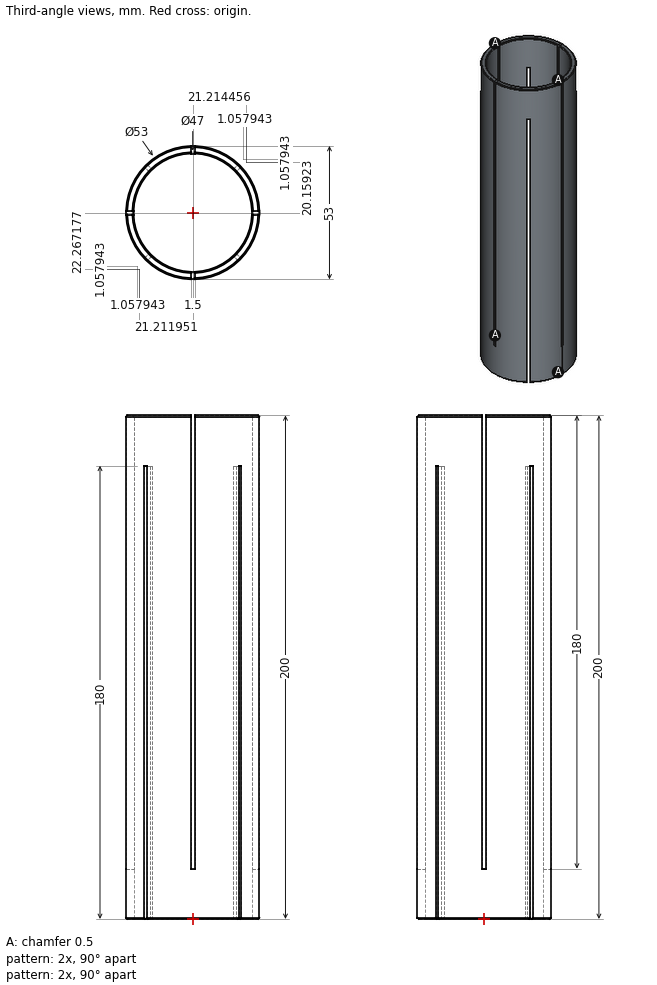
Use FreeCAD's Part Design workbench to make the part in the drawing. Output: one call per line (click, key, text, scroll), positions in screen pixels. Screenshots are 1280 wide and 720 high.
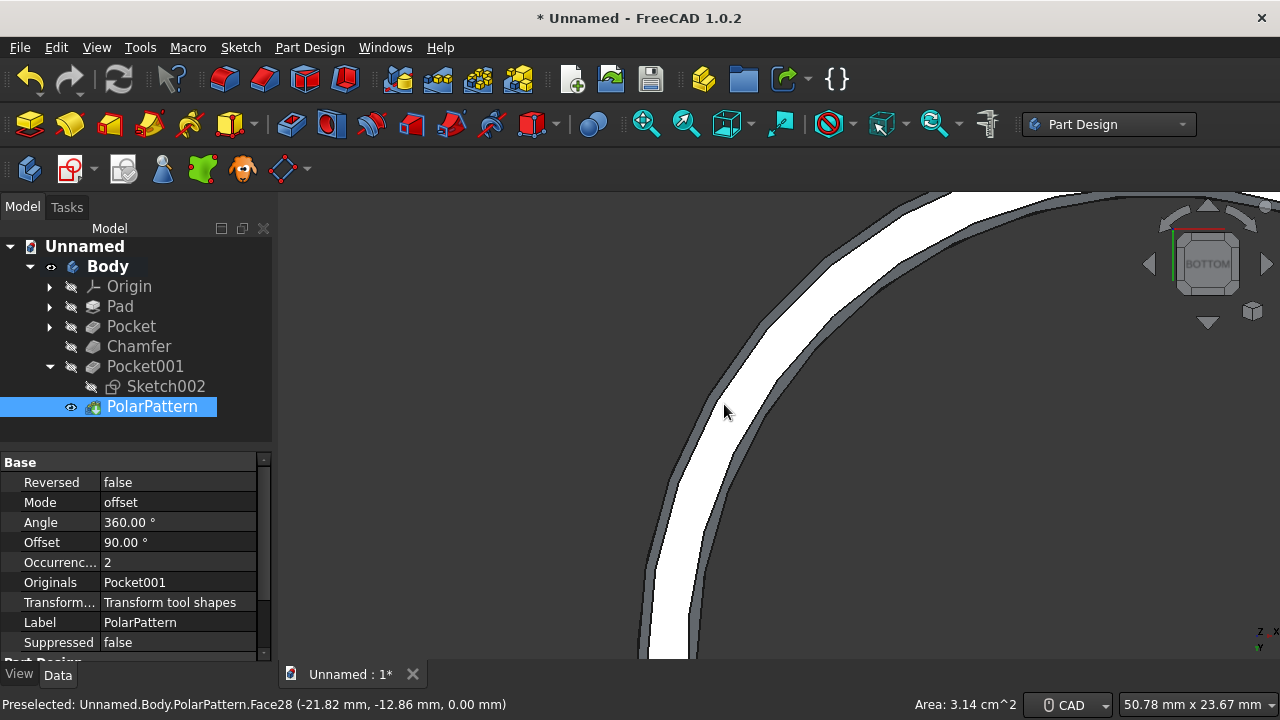
click(70, 170)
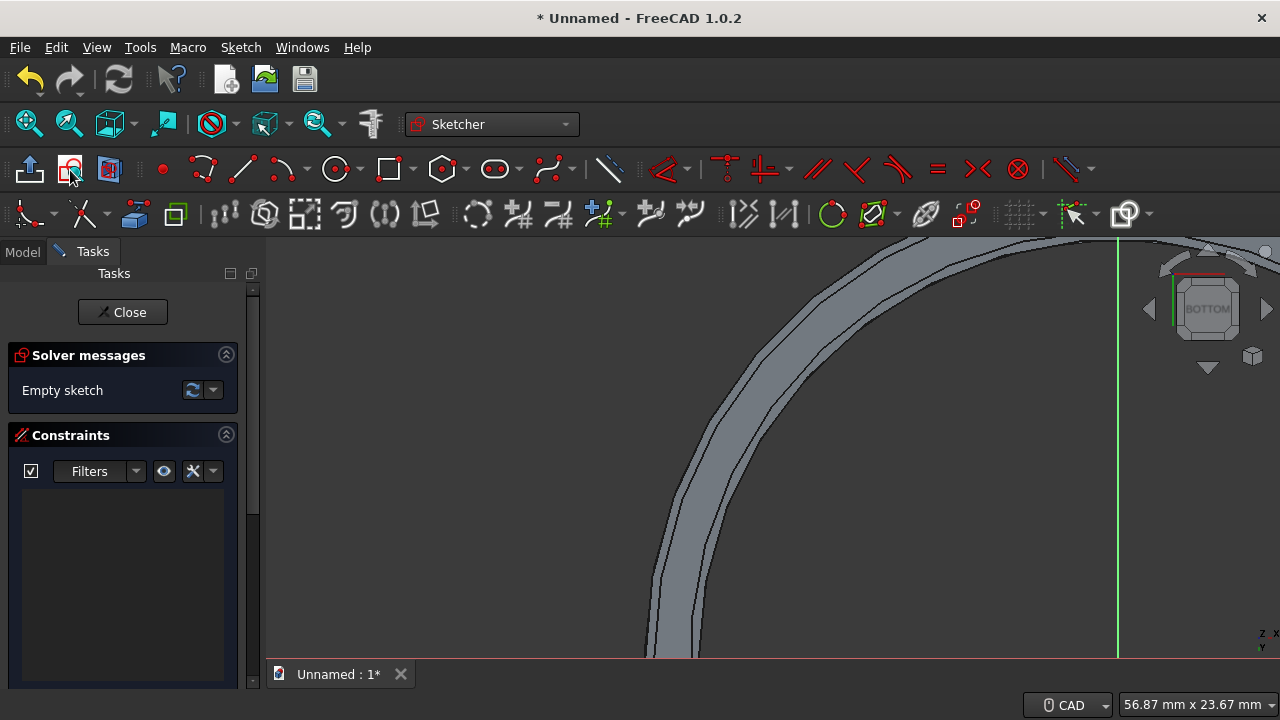
scroll(469, 331, down, 5)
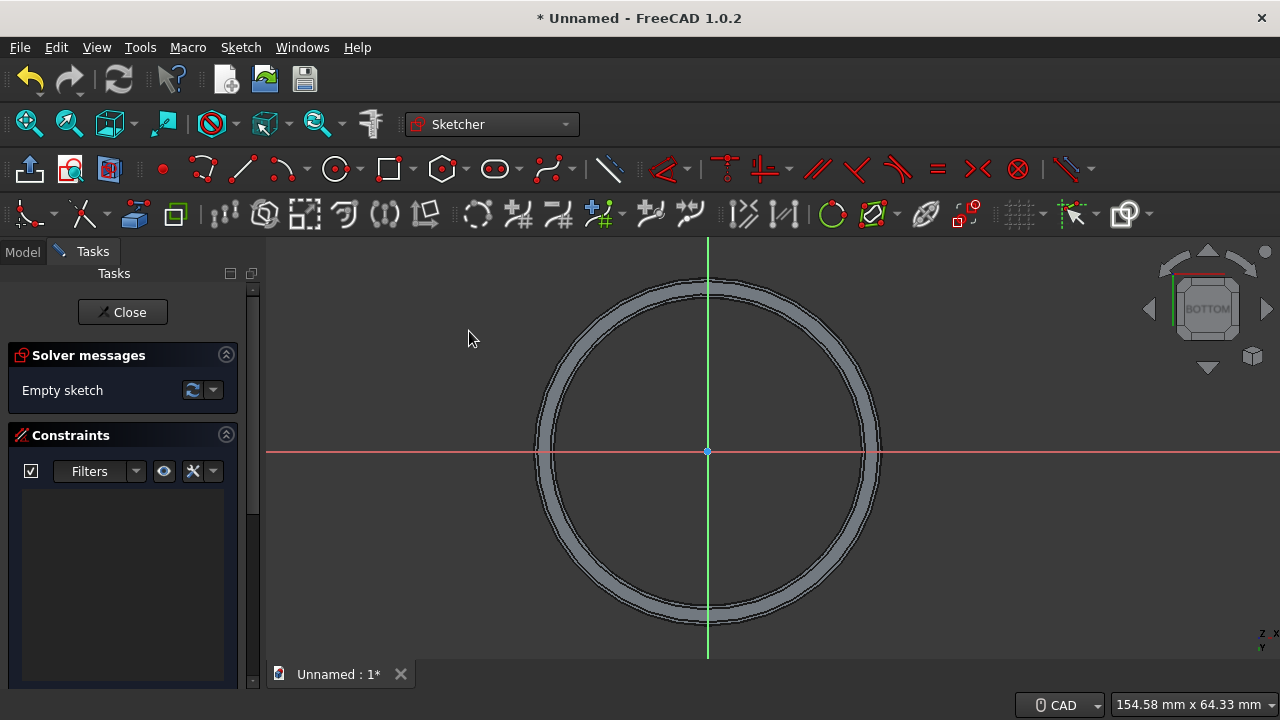
click(204, 170)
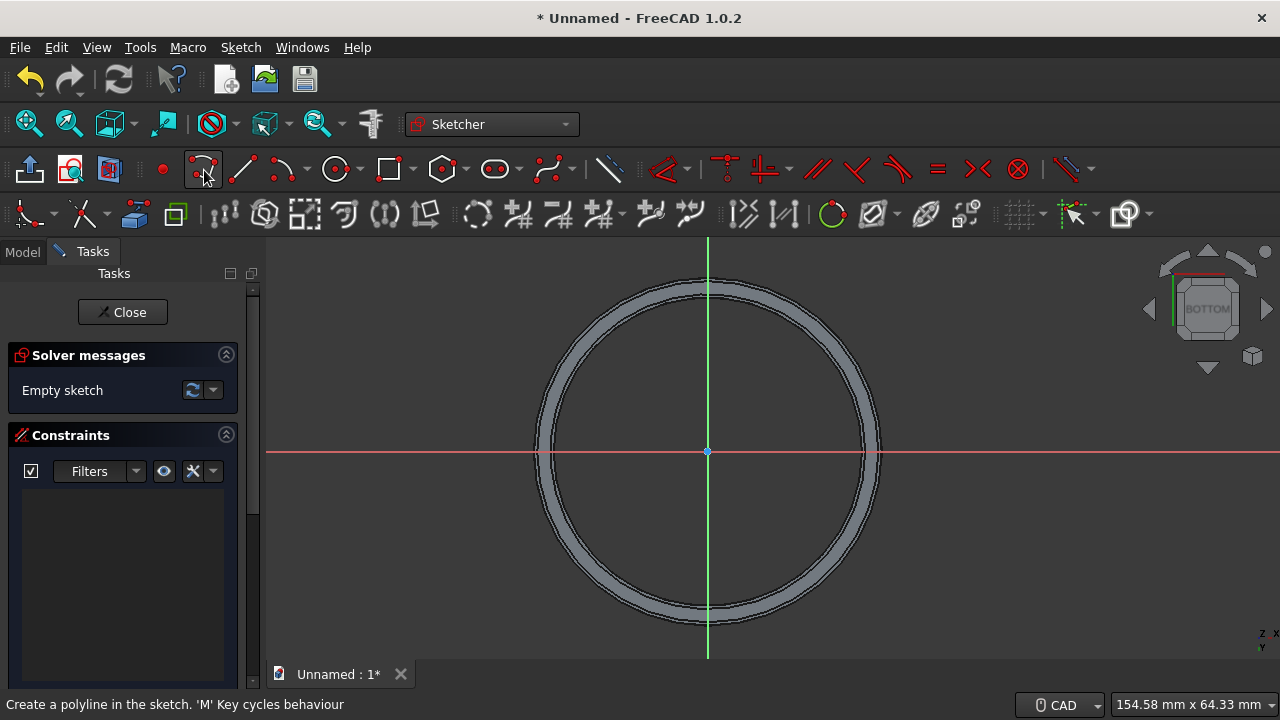
click(847, 584)
click(569, 306)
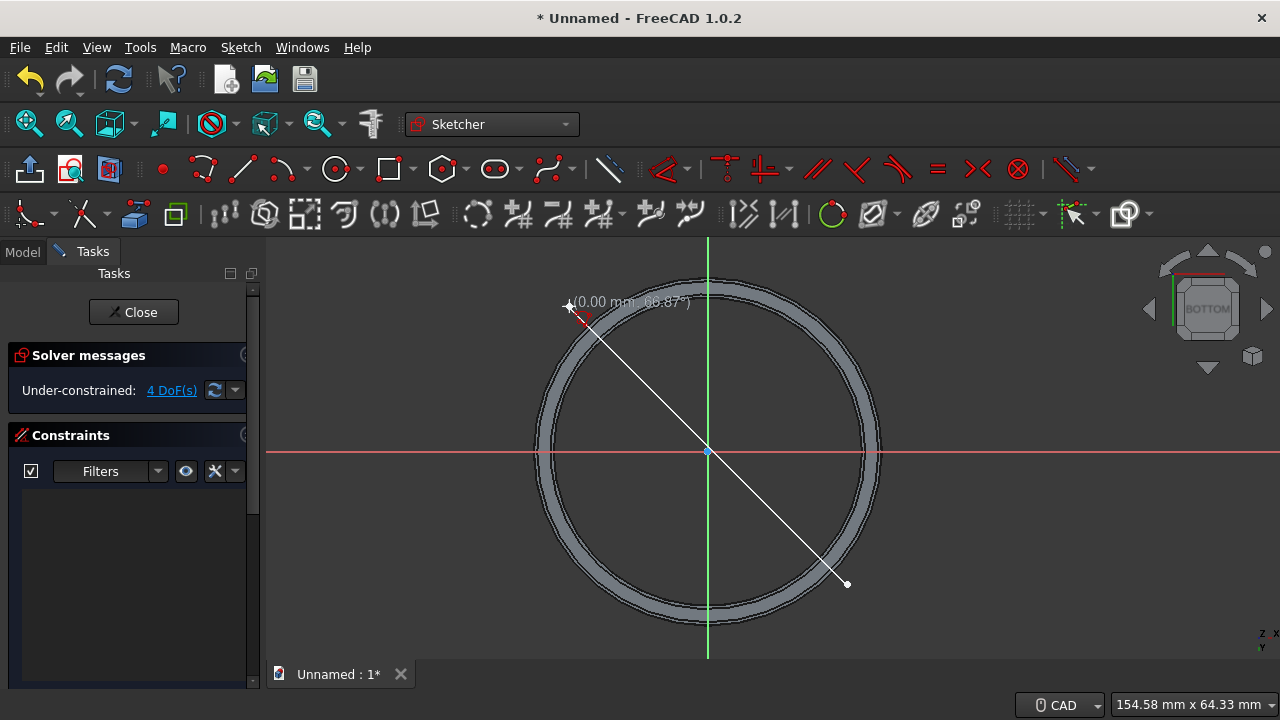
scroll(562, 313, up, 3)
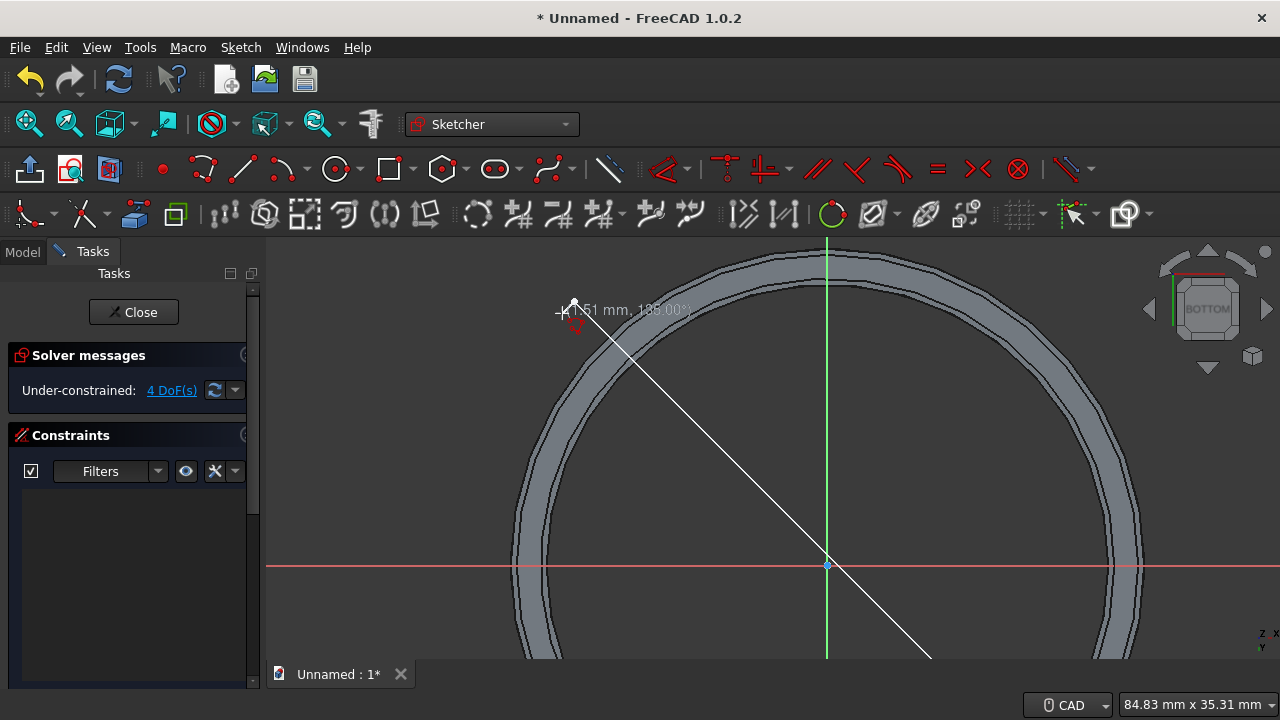
click(561, 312)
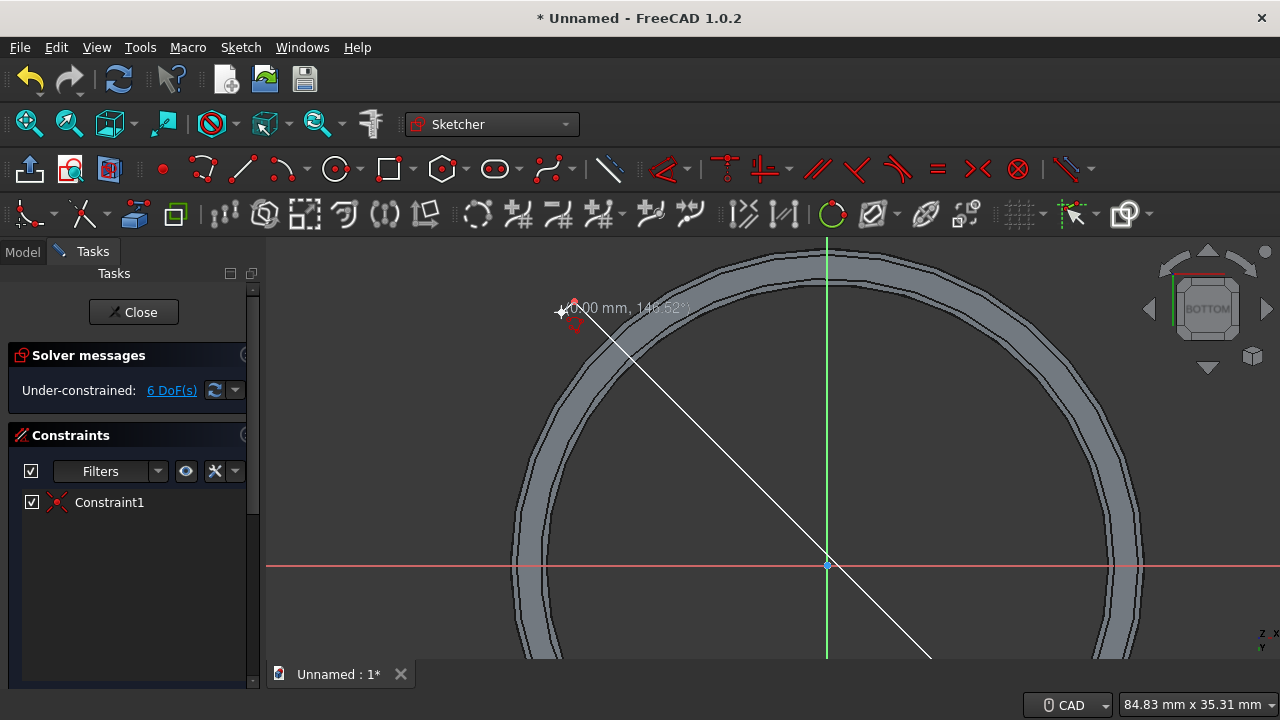
scroll(563, 313, down, 3)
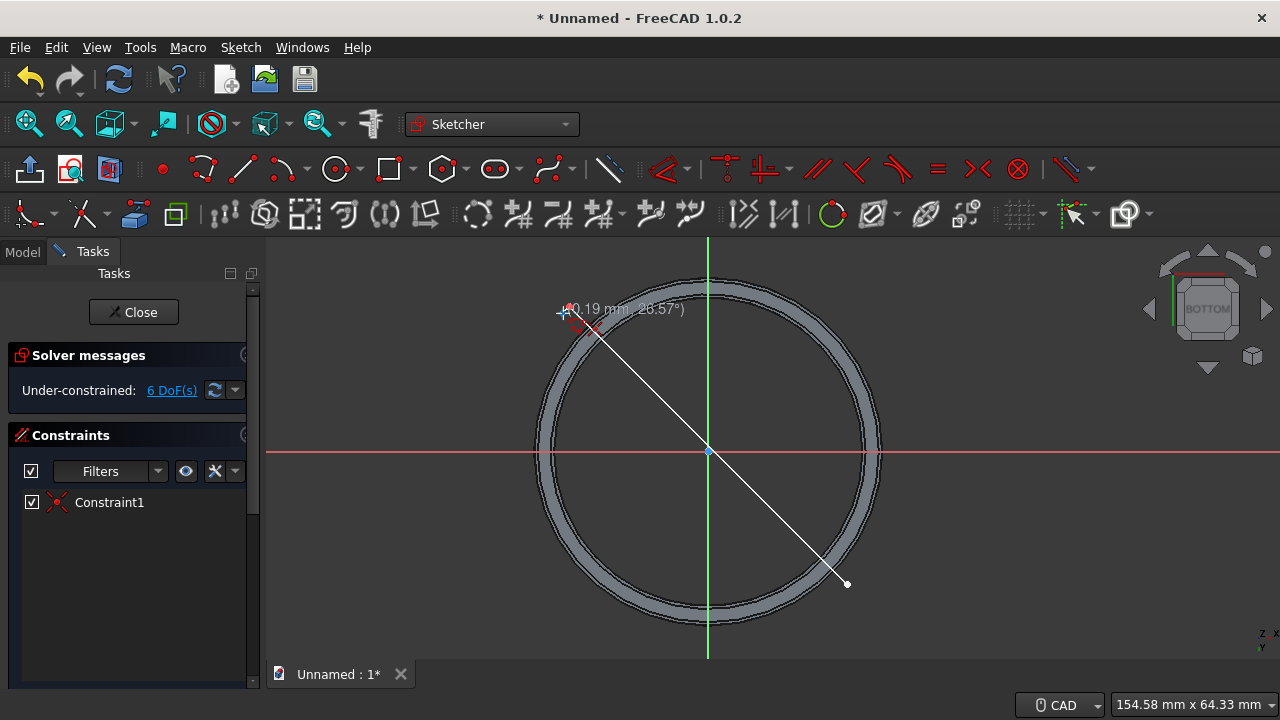
scroll(840, 591, up, 3)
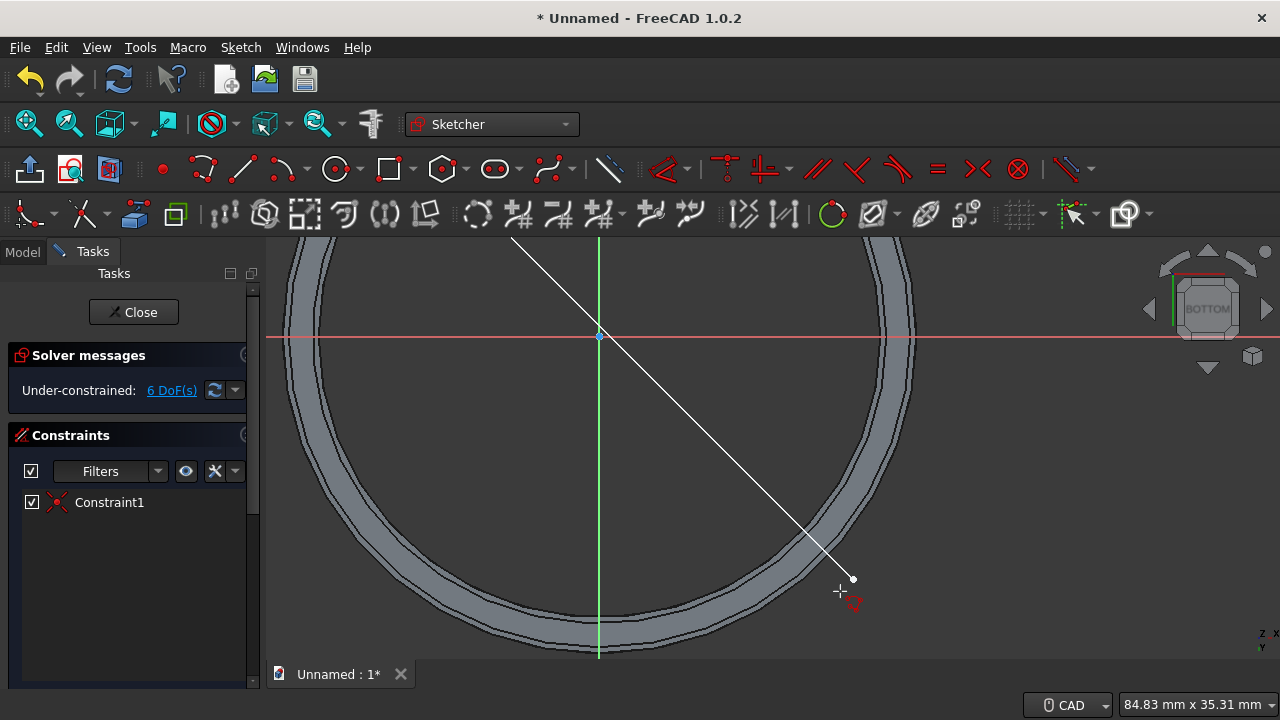
click(840, 590)
click(853, 579)
key(Escape)
key(Escape)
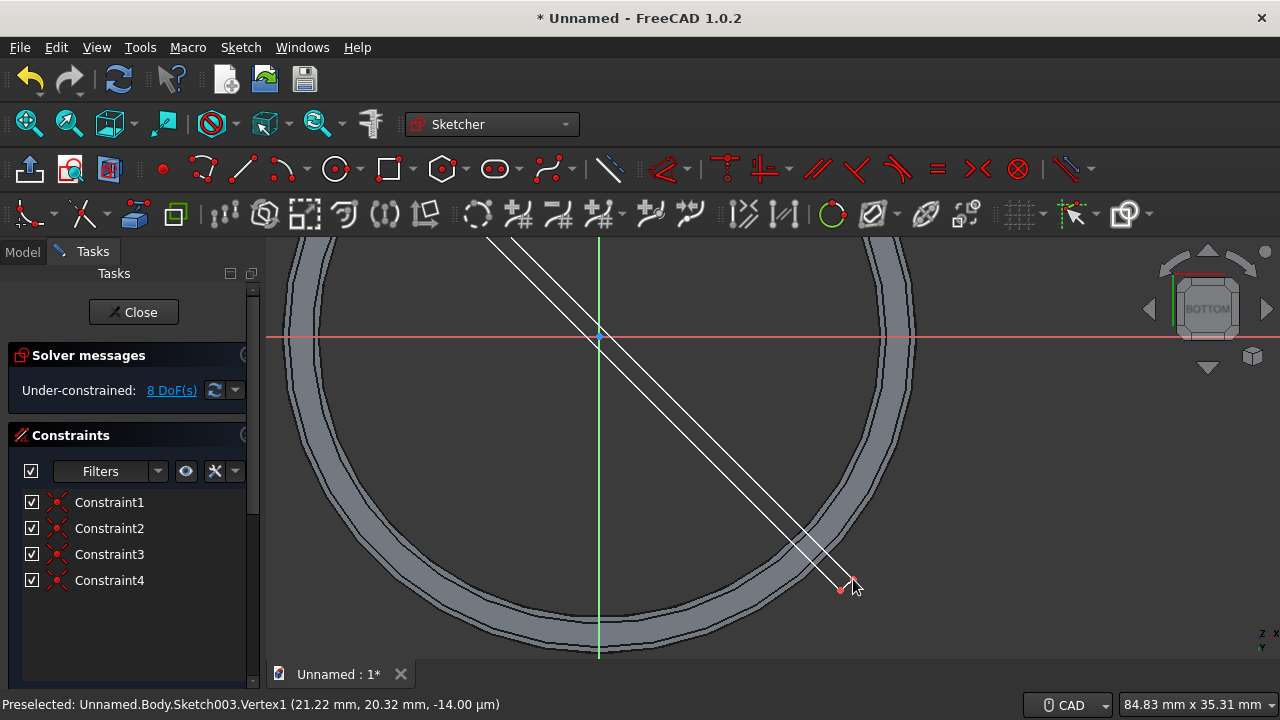
click(664, 170)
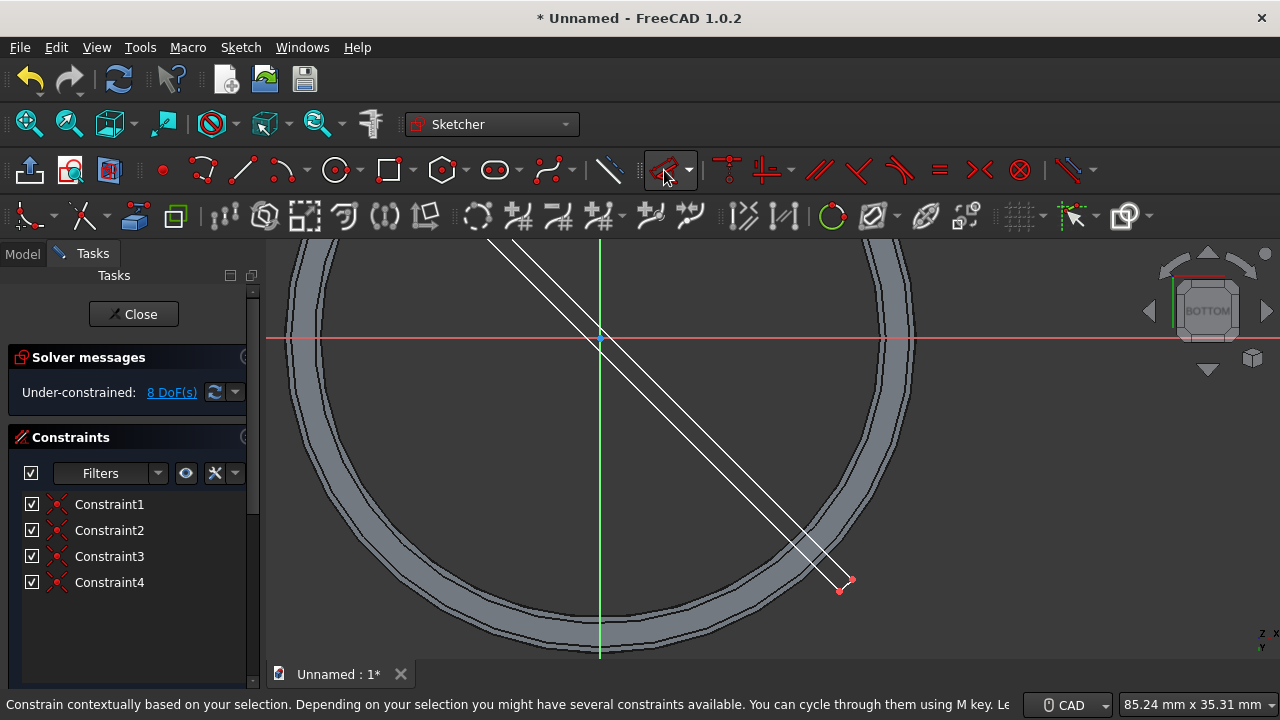
click(853, 580)
click(887, 459)